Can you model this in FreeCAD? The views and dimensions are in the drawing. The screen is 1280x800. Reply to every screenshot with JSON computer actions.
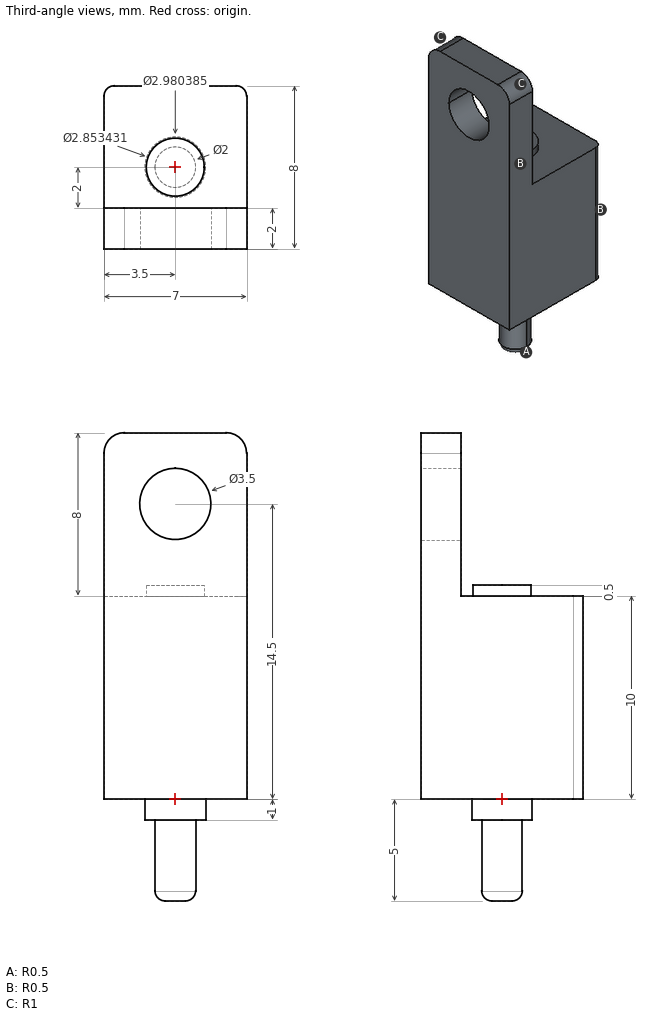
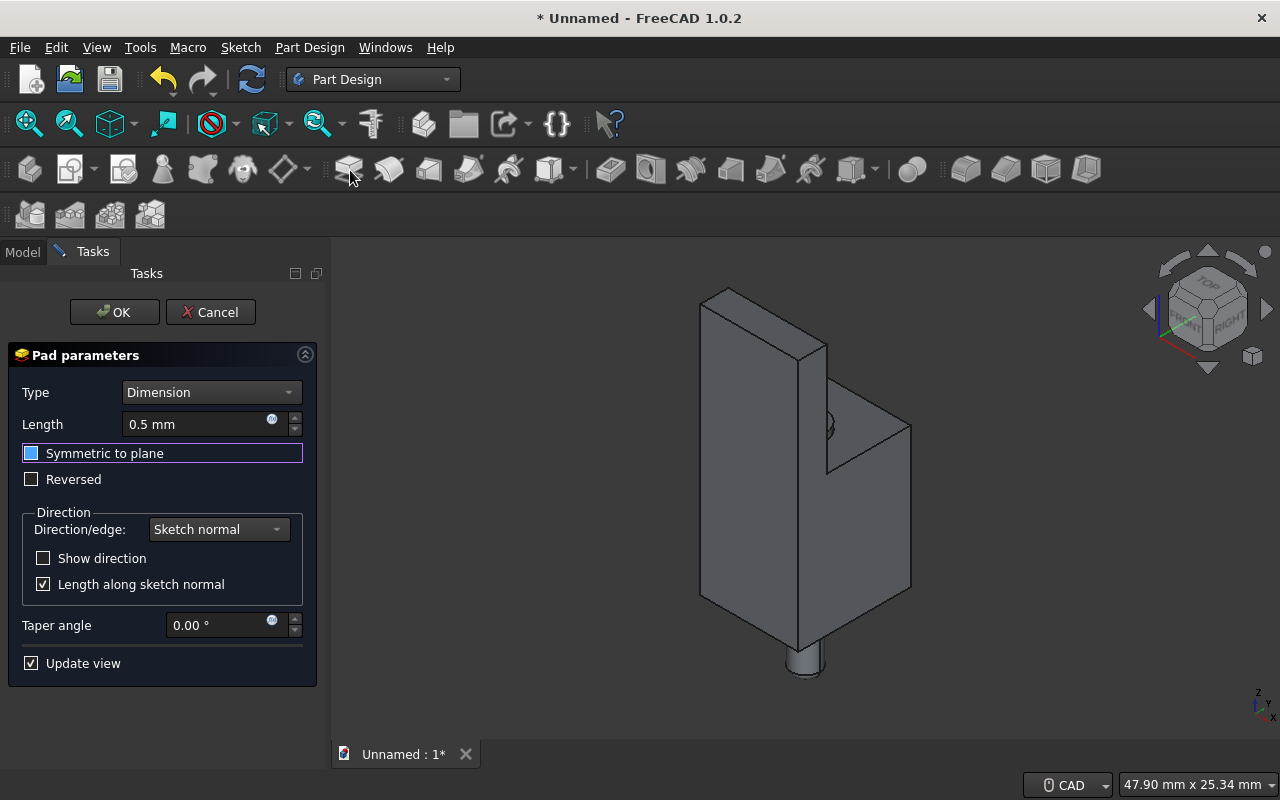
{"action": "left_click", "coordinate": [115, 312]}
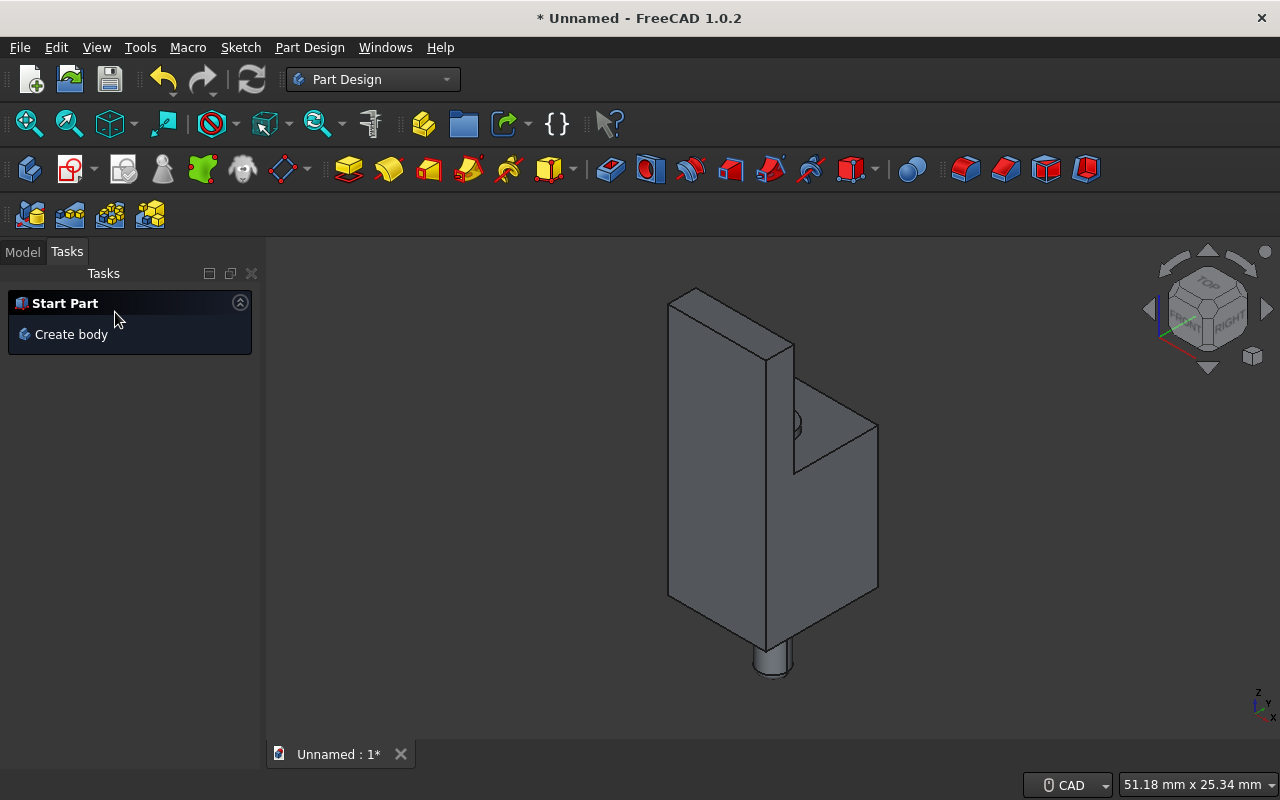
{"action": "key", "text": "2"}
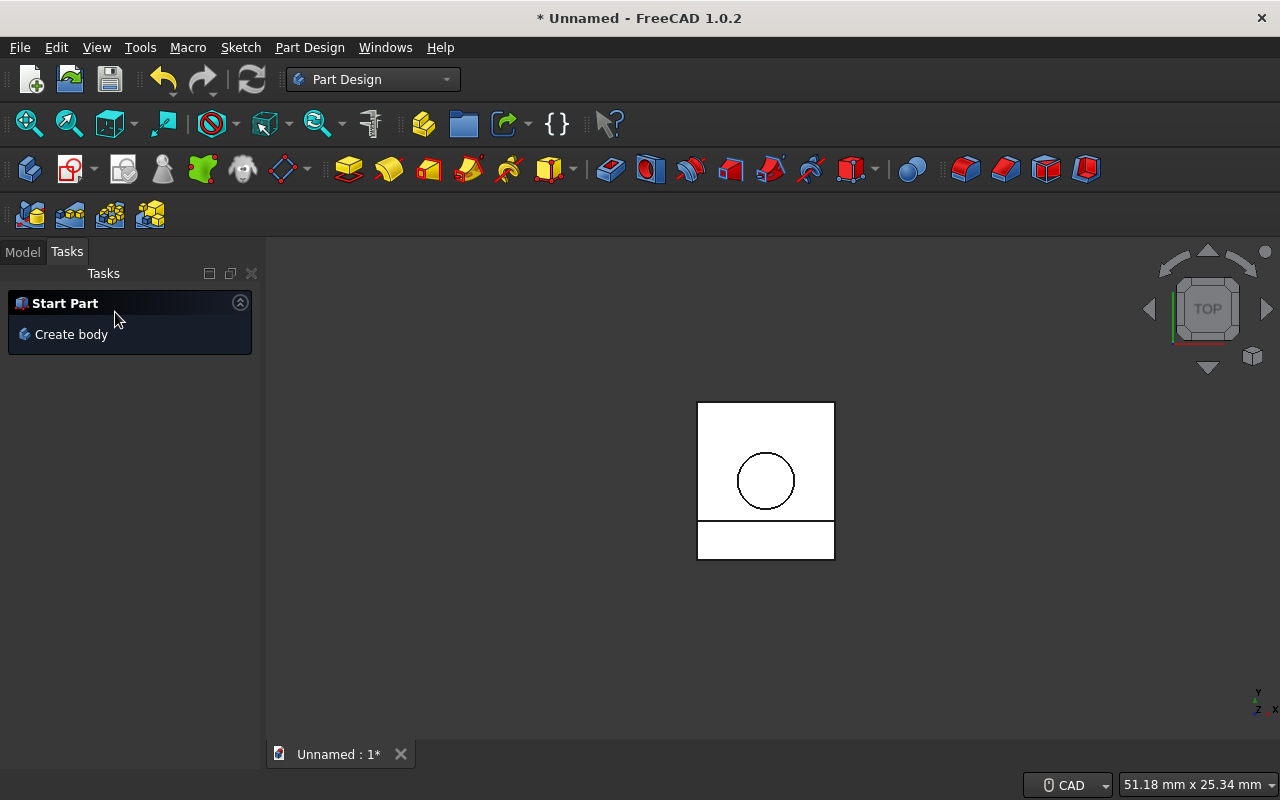
{"action": "key", "text": "v f"}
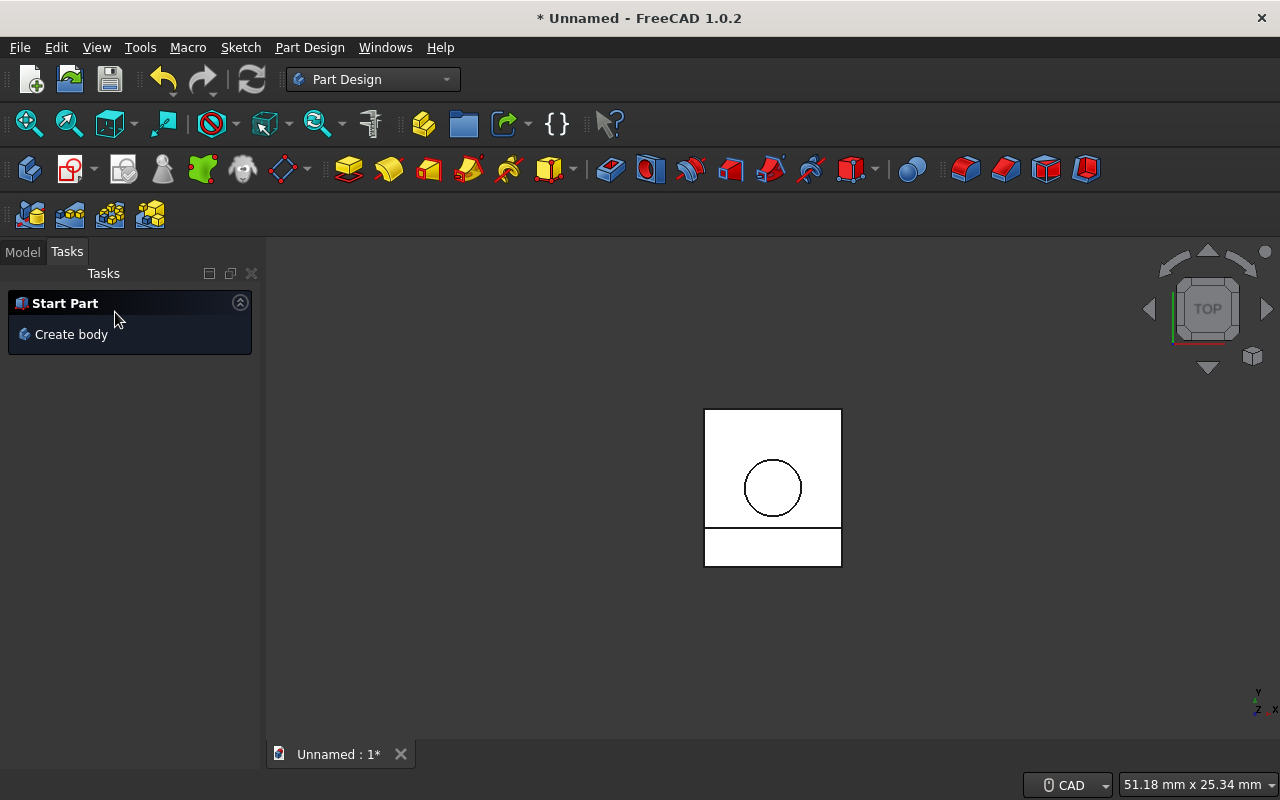
{"action": "key", "text": "0"}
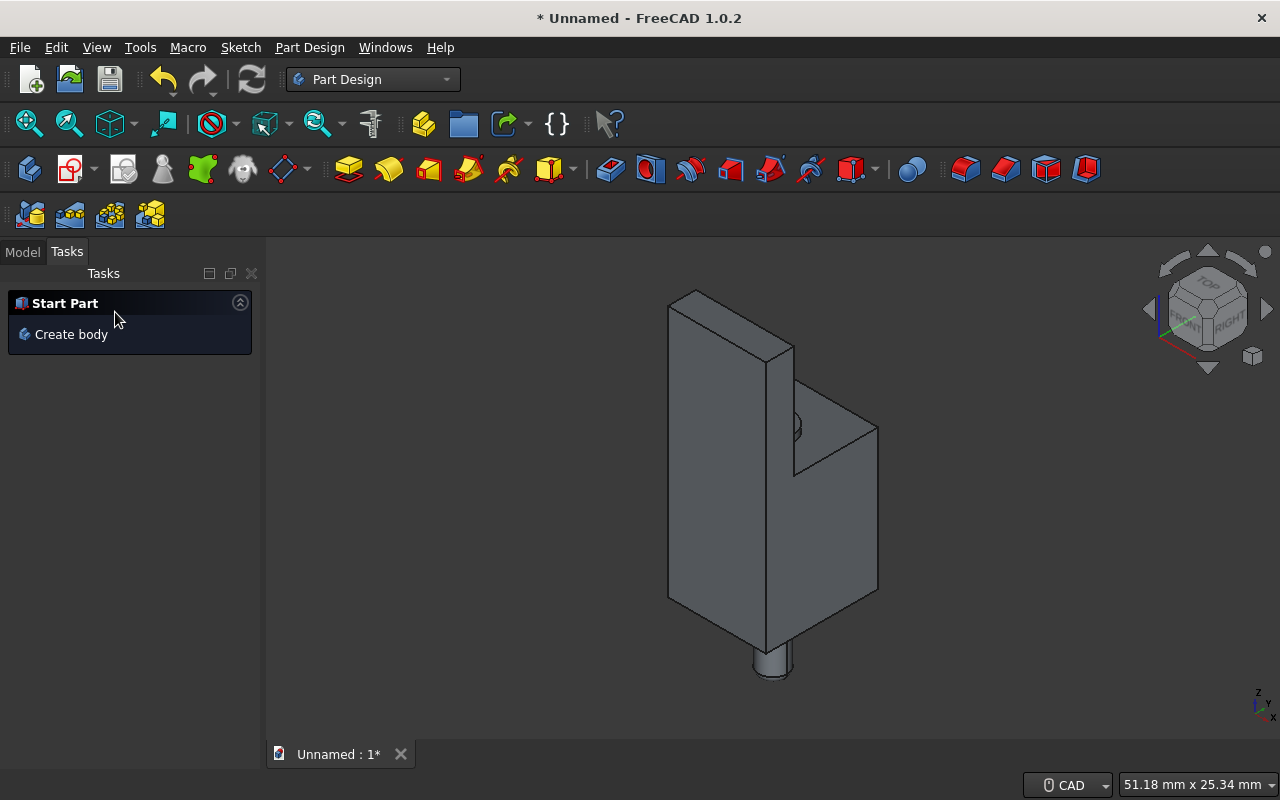
{"action": "key", "text": "1"}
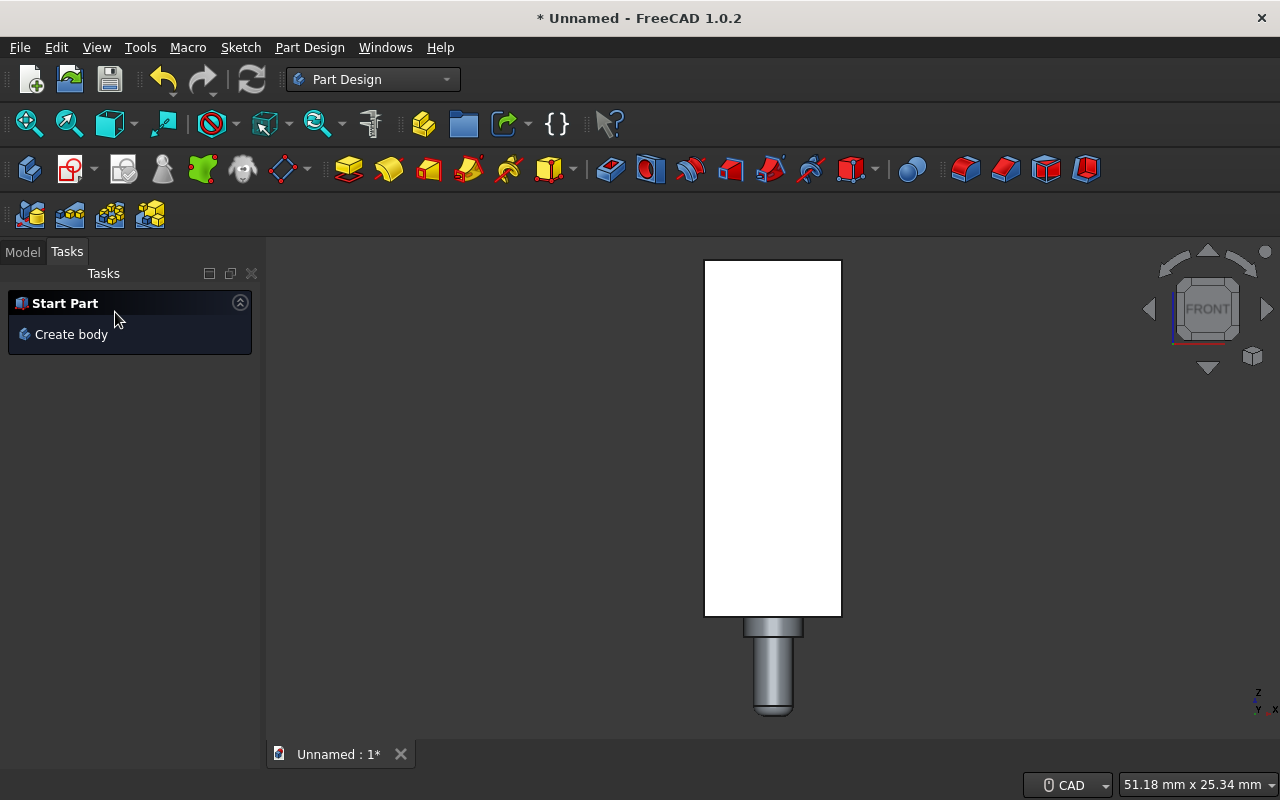
{"action": "key", "text": "3"}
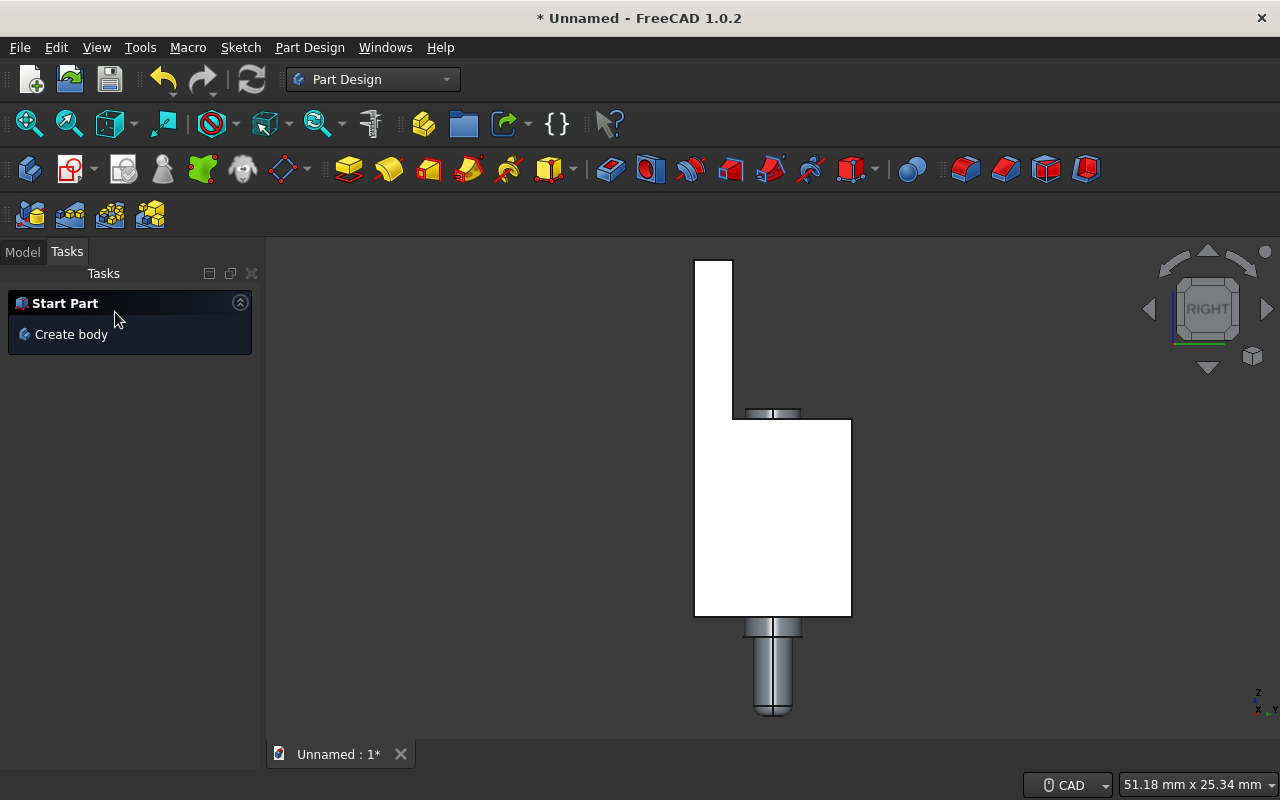
{"action": "left_click", "coordinate": [852, 517]}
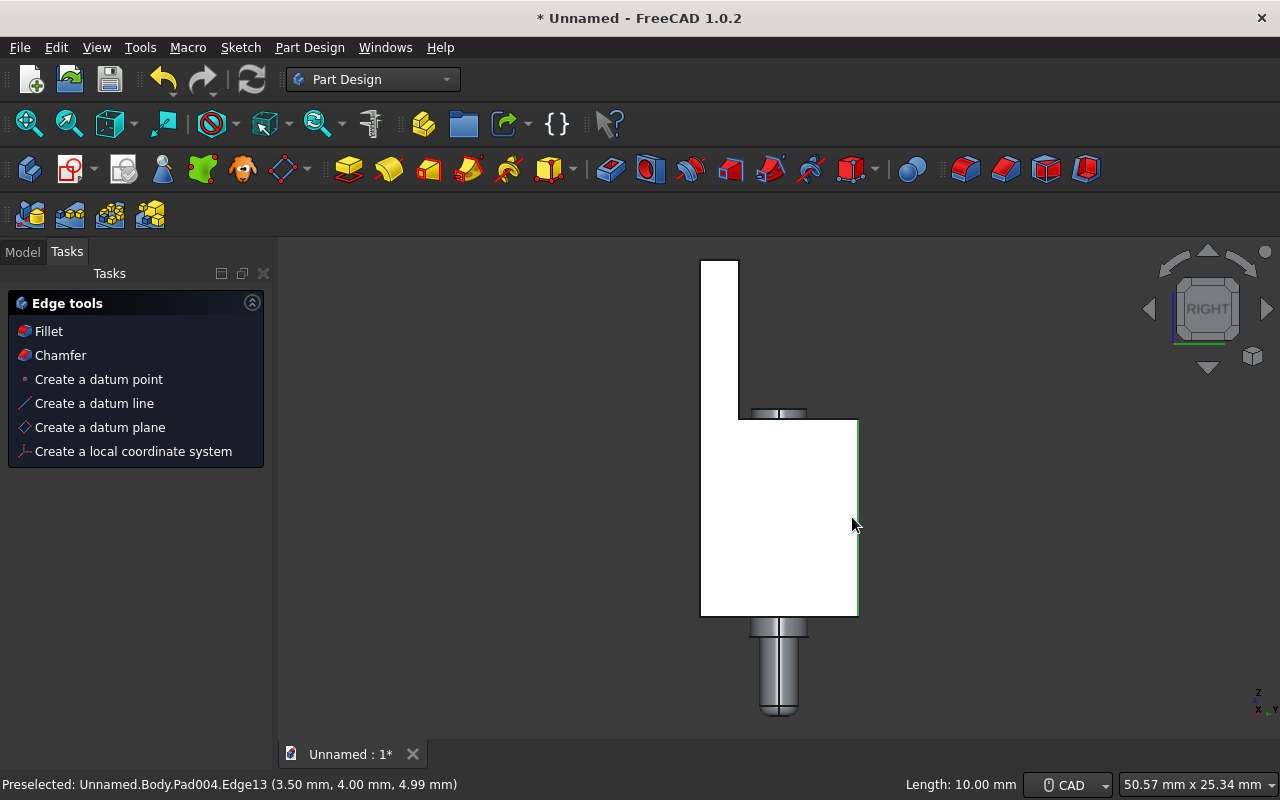
{"action": "key", "text": "5"}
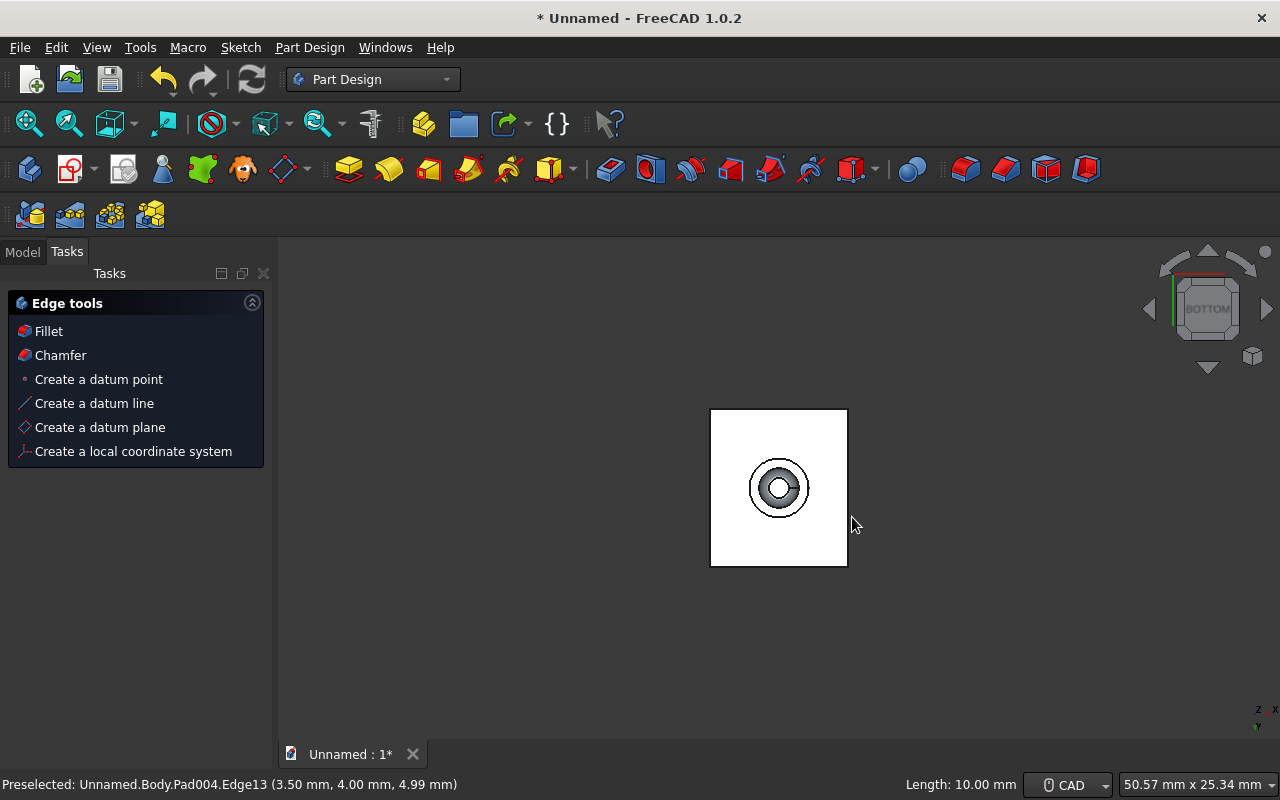
{"action": "key", "text": "v f"}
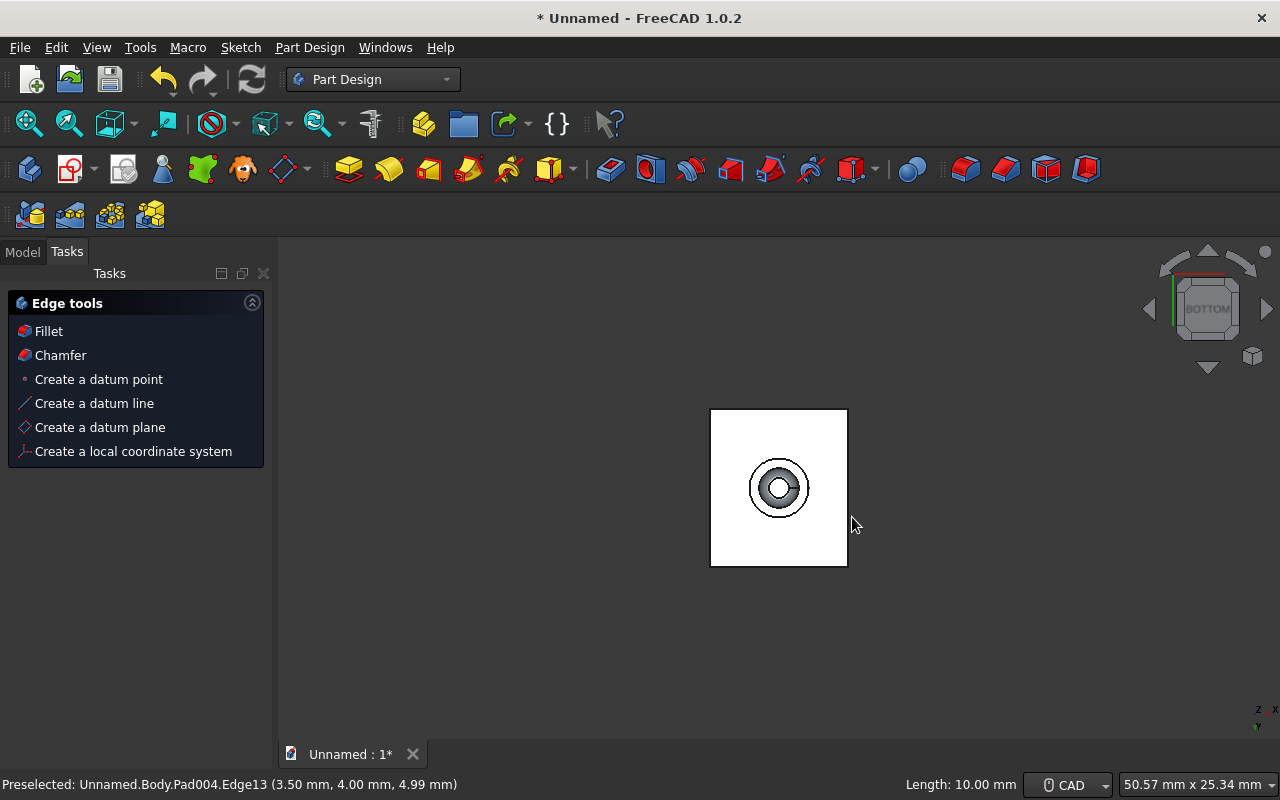
{"action": "key", "text": "4"}